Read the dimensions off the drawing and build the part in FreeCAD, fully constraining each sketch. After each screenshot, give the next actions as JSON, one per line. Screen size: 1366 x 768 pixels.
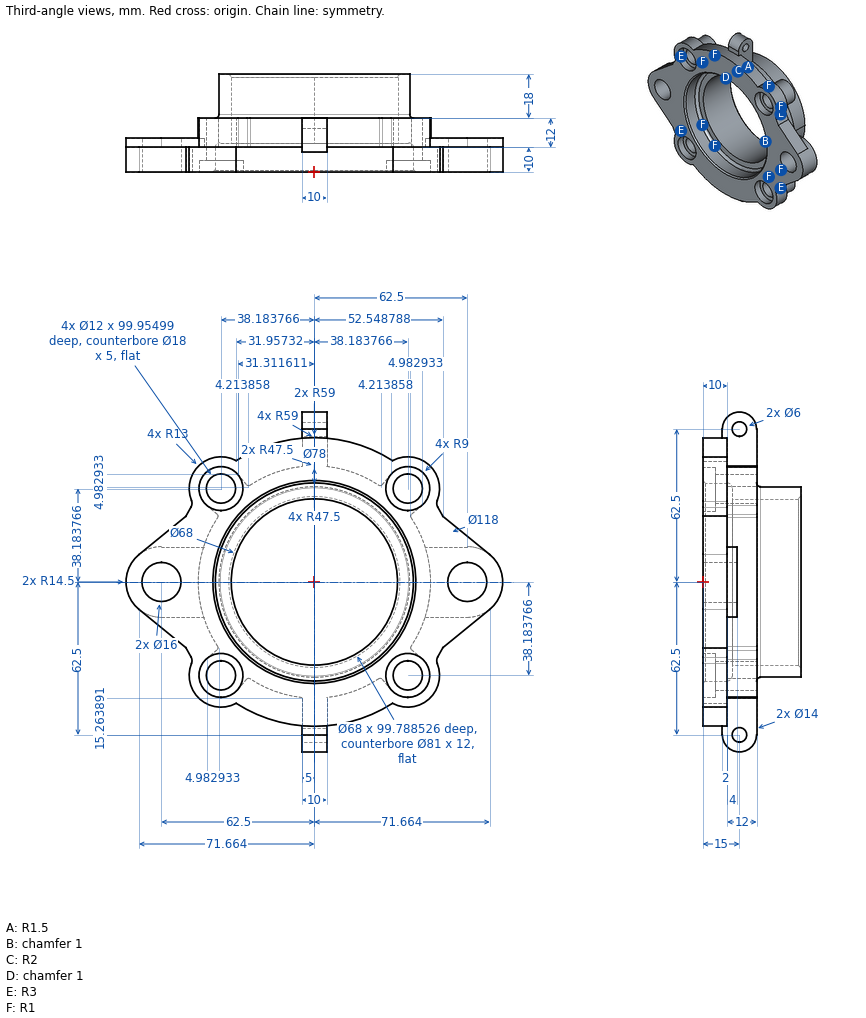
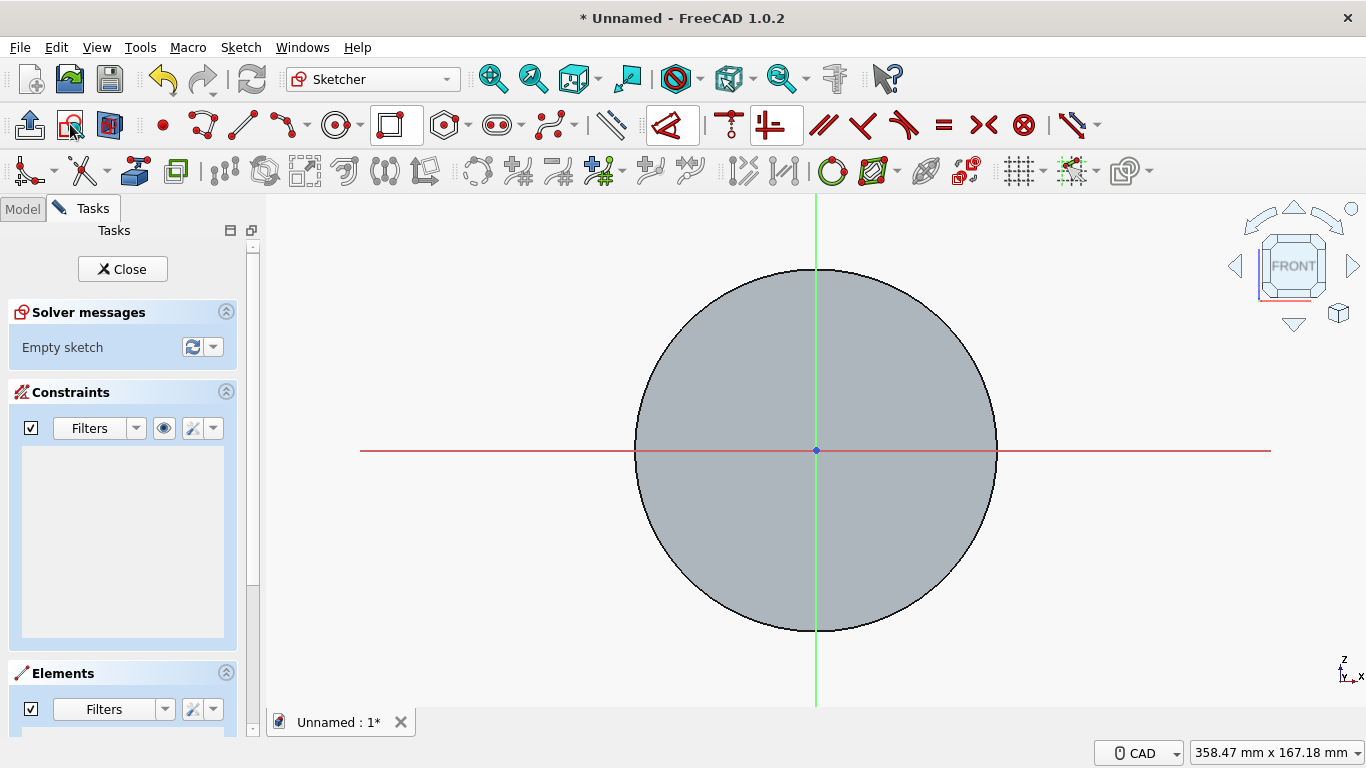
{"action": "left_click", "coordinate": [244, 126]}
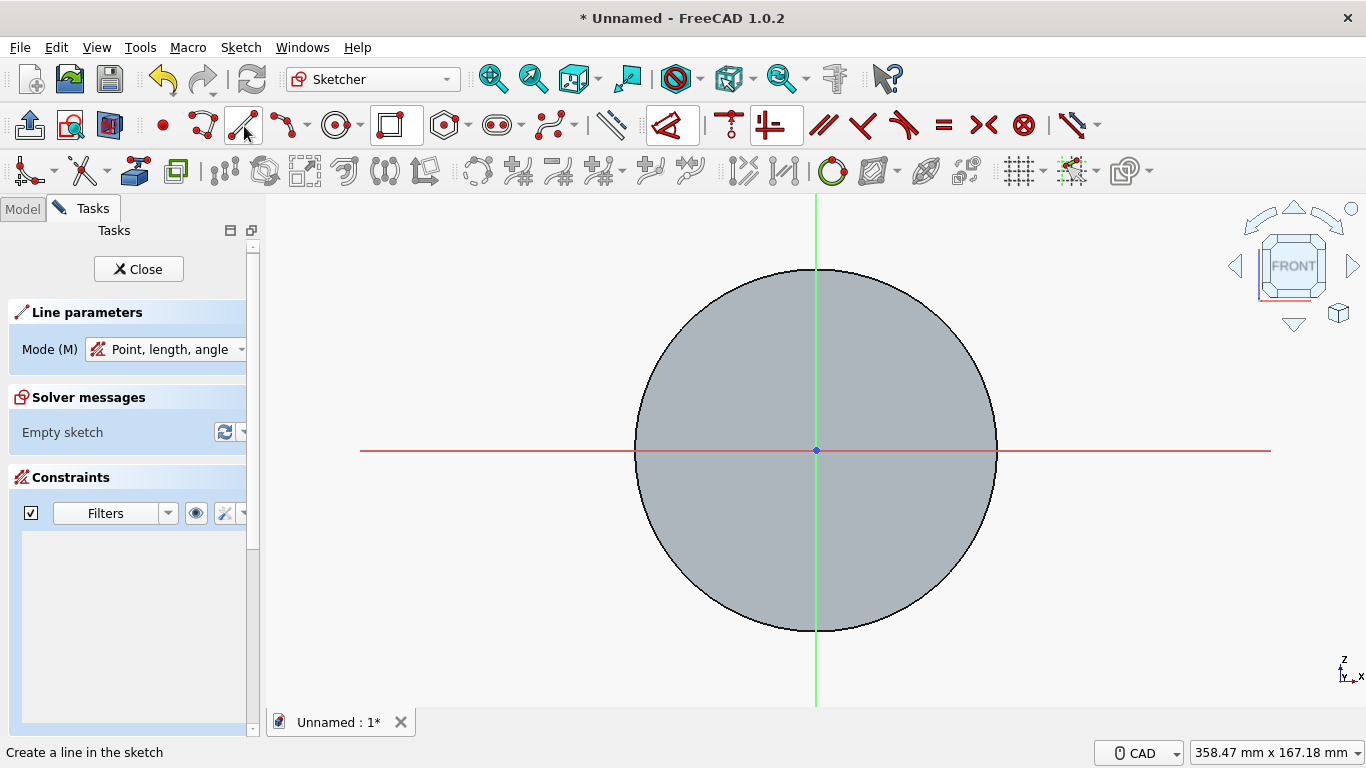
{"action": "left_click", "coordinate": [1036, 416]}
{"action": "left_click", "coordinate": [977, 368]}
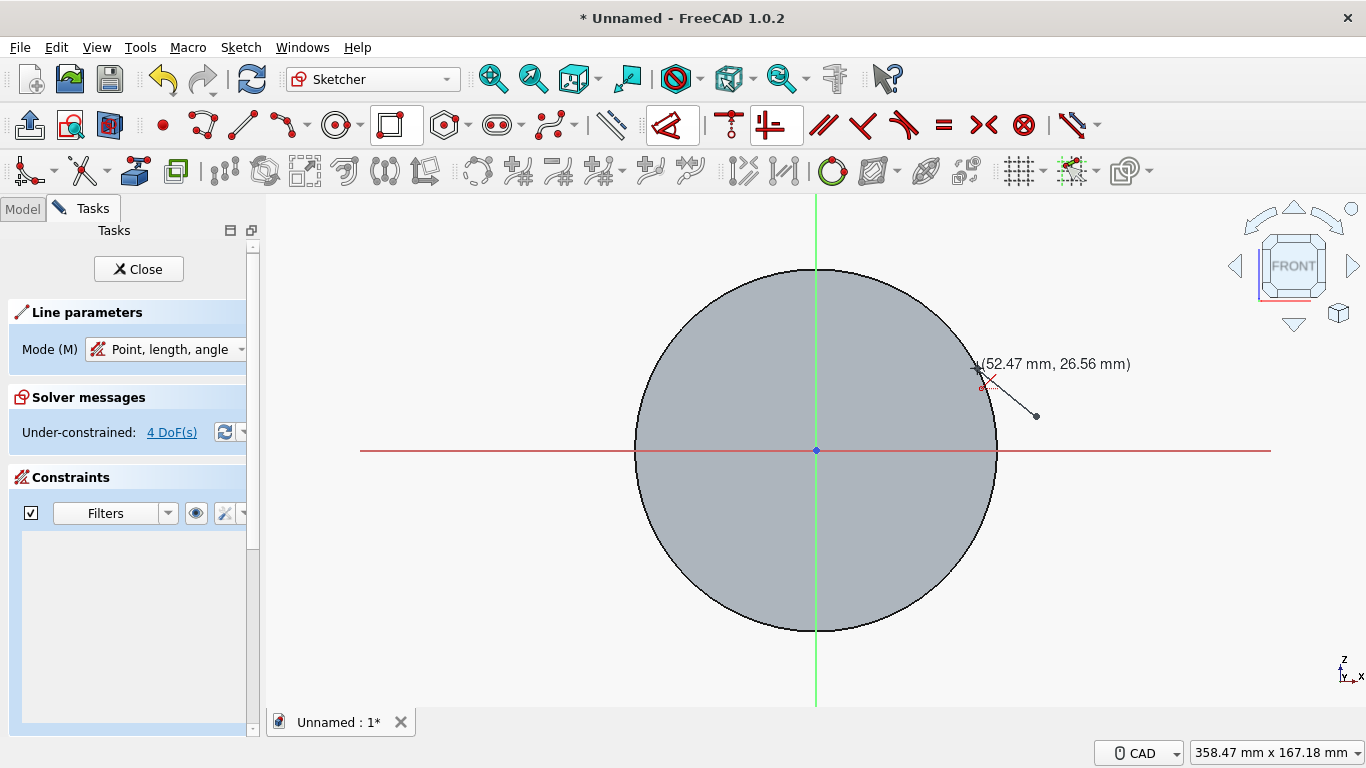
{"action": "left_click", "coordinate": [655, 368]}
{"action": "left_click", "coordinate": [596, 416]}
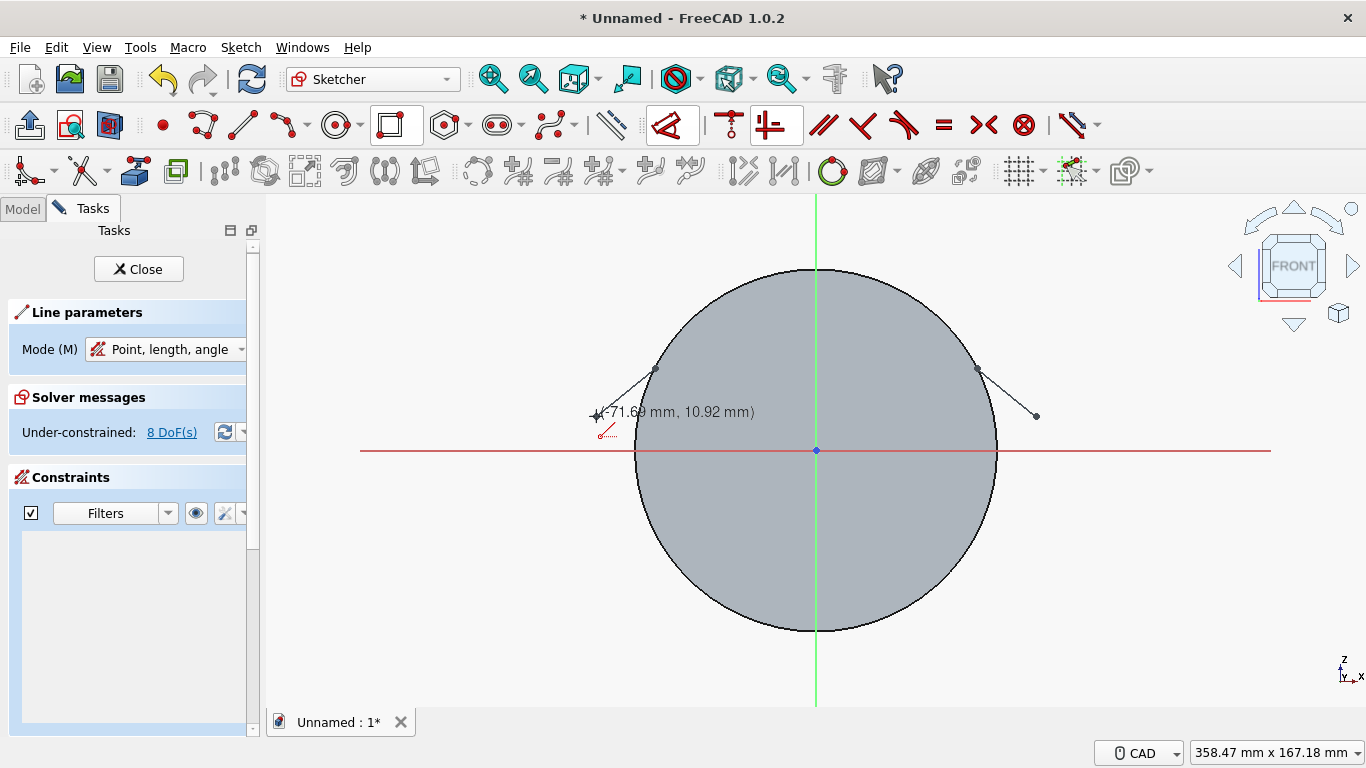
{"action": "left_click", "coordinate": [596, 485]}
{"action": "left_click", "coordinate": [655, 533]}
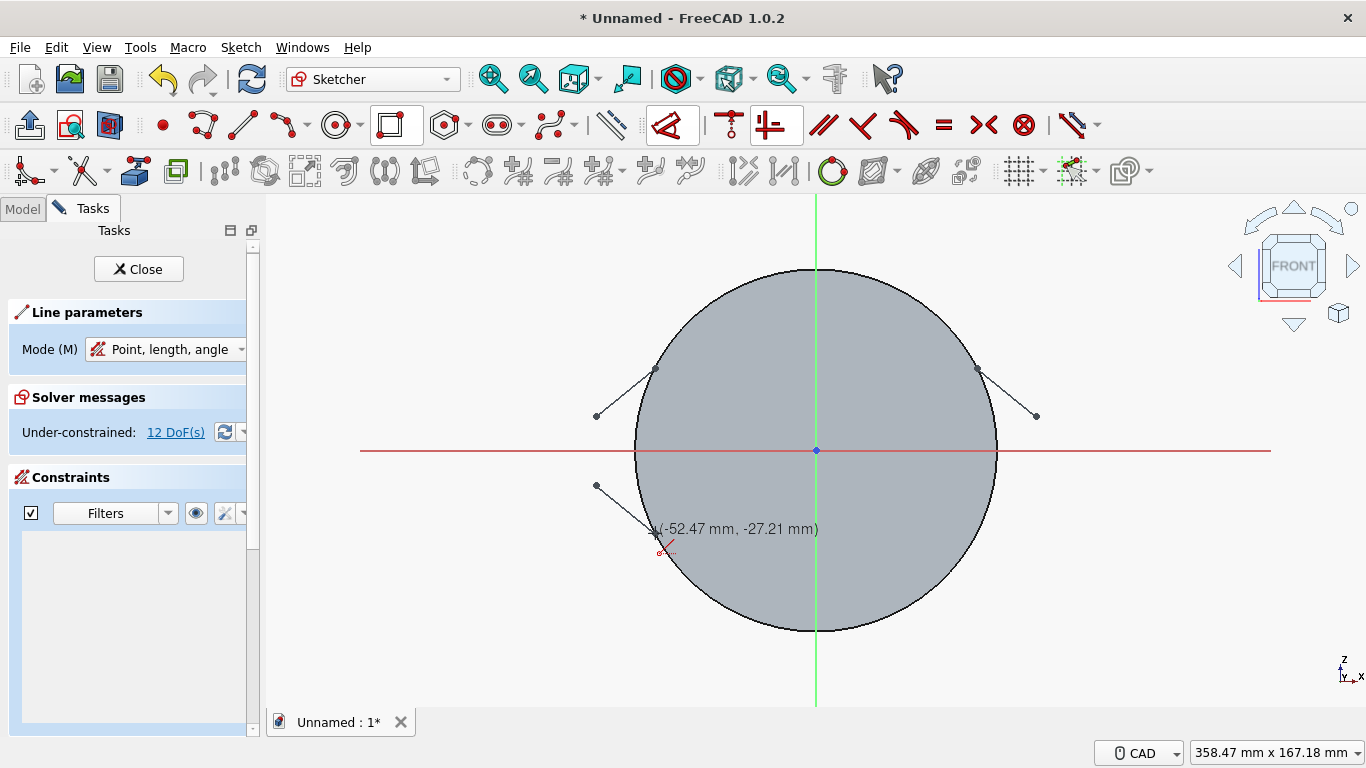
{"action": "left_click", "coordinate": [977, 533]}
{"action": "left_click", "coordinate": [1036, 485]}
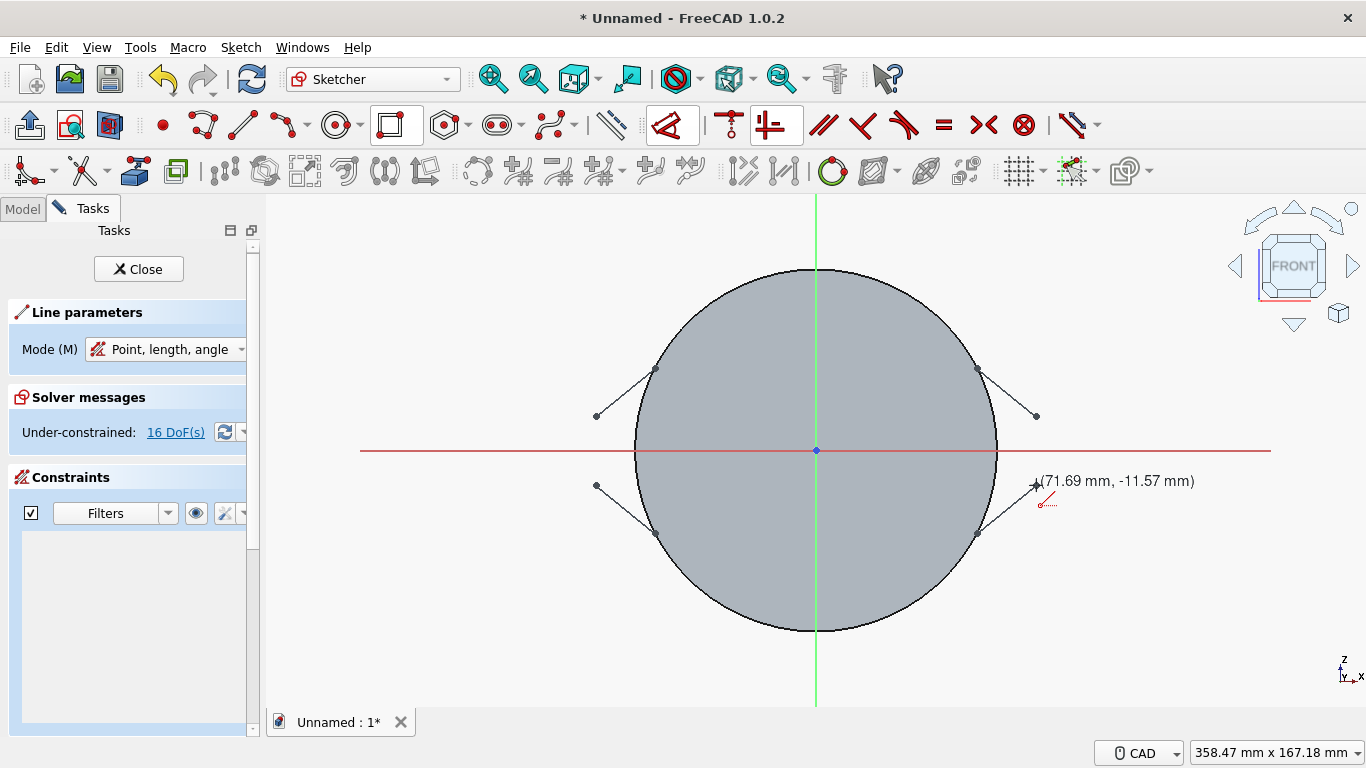
{"action": "left_click", "coordinate": [284, 126]}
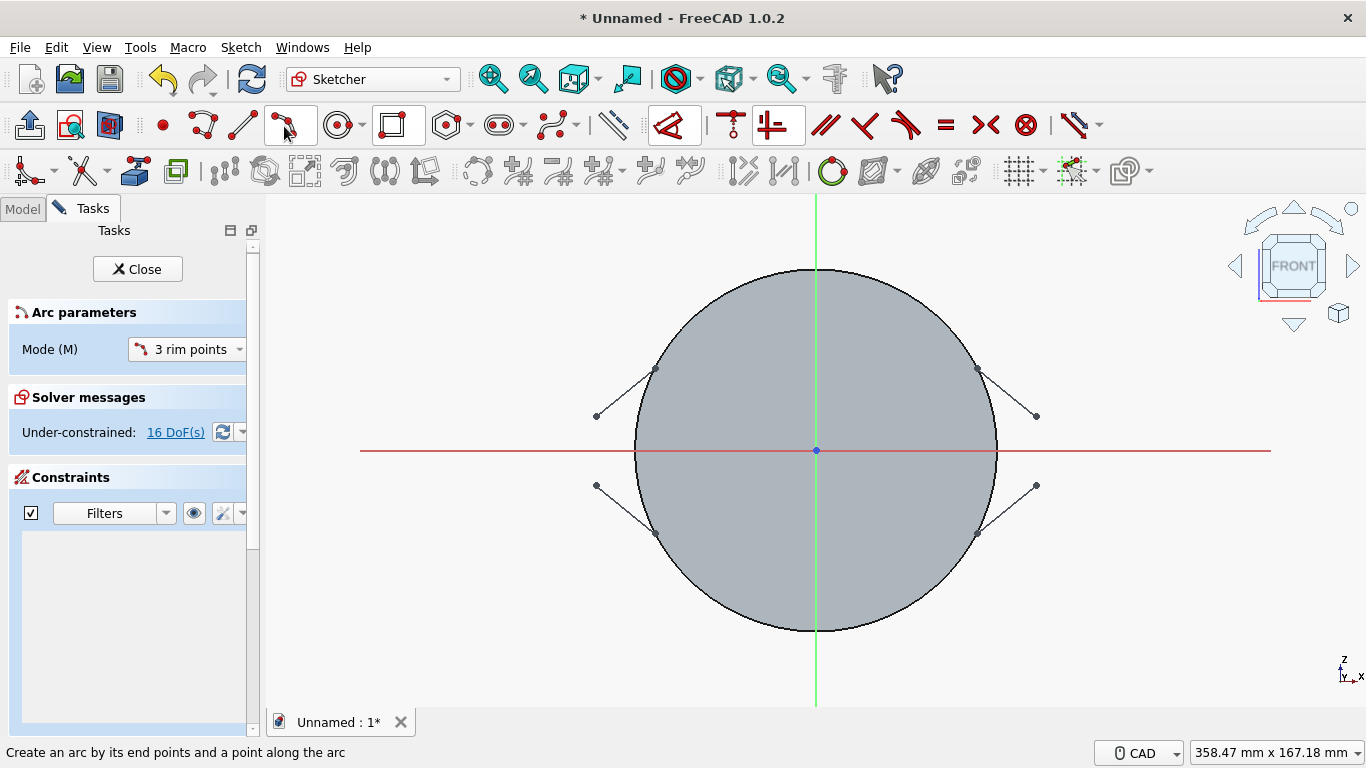
{"action": "left_click", "coordinate": [977, 369]}
{"action": "left_click", "coordinate": [655, 369]}
{"action": "left_click", "coordinate": [855, 274]}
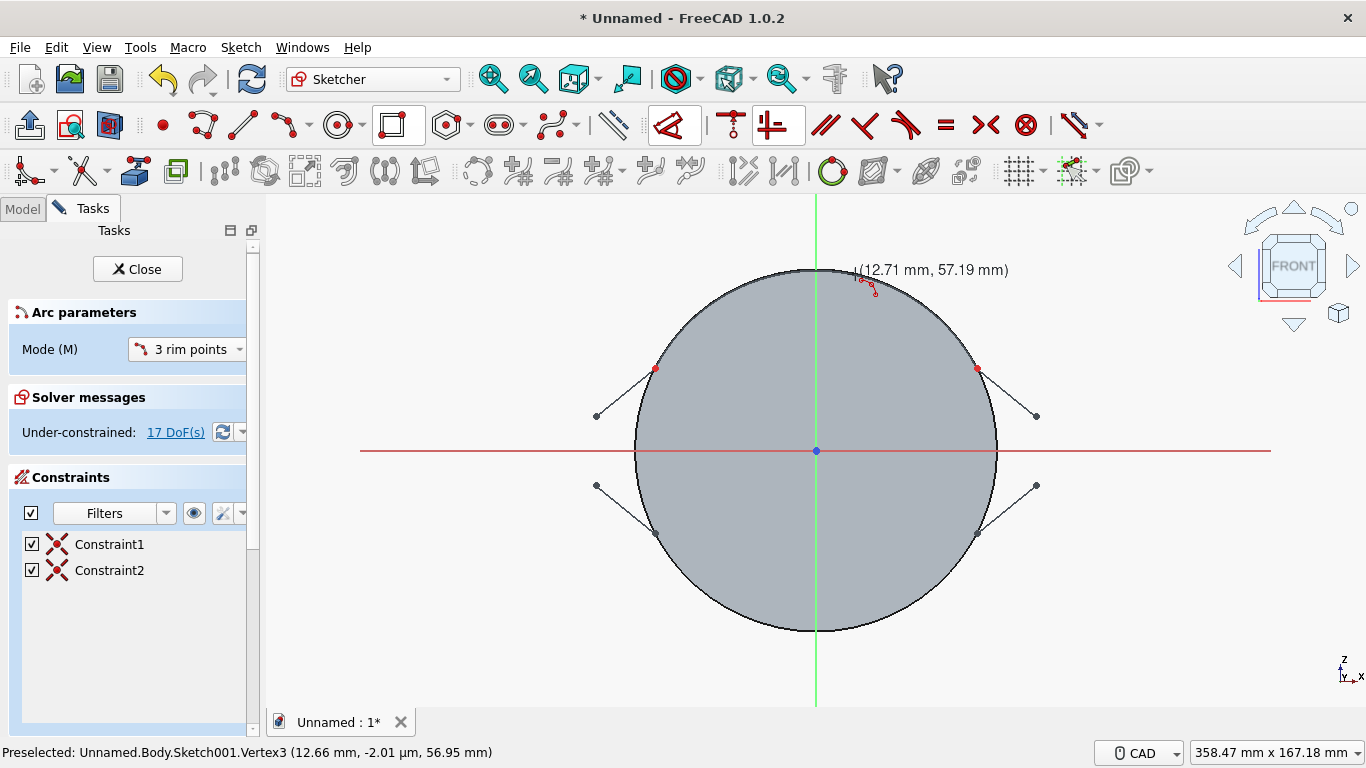
{"action": "left_click", "coordinate": [596, 417]}
{"action": "left_click", "coordinate": [596, 486]}
{"action": "left_click", "coordinate": [582, 435]}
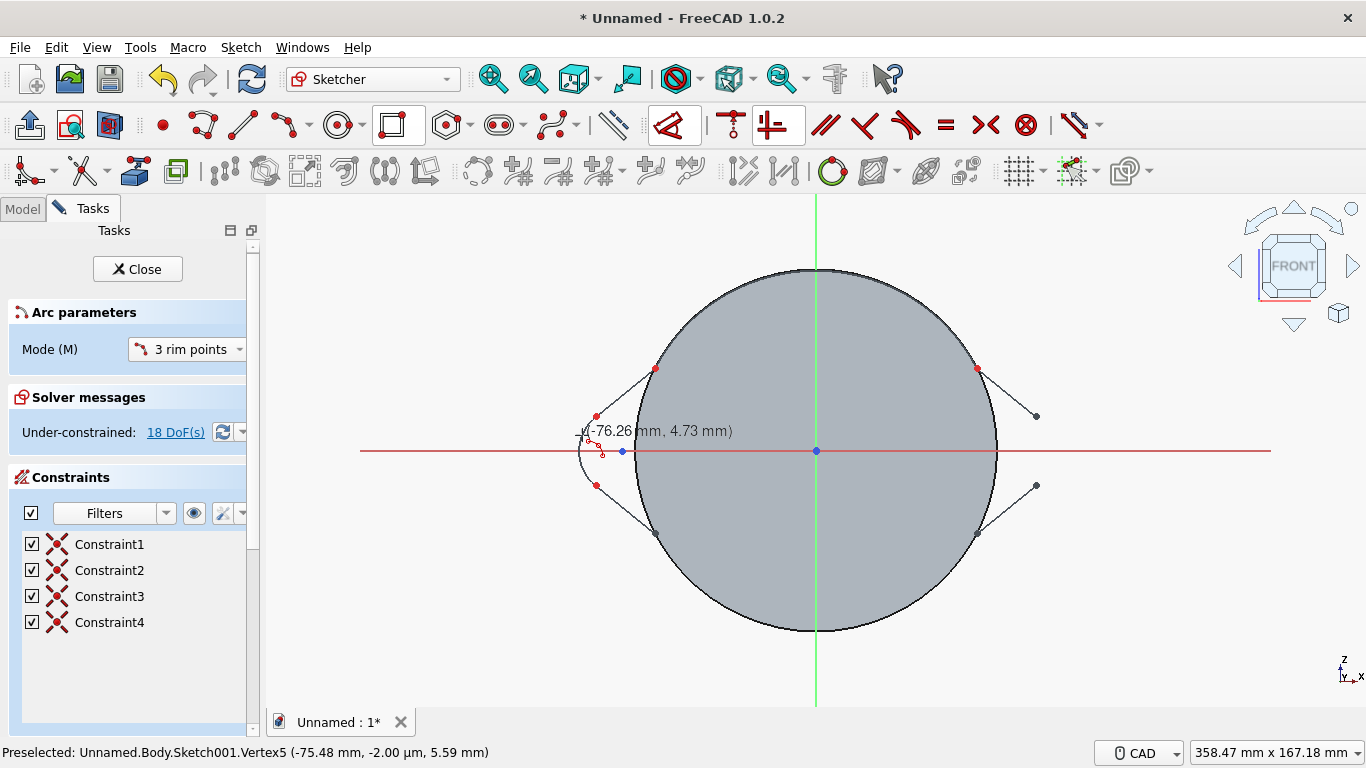
{"action": "left_click", "coordinate": [655, 534]}
{"action": "left_click", "coordinate": [977, 534]}
{"action": "left_click", "coordinate": [777, 627]}